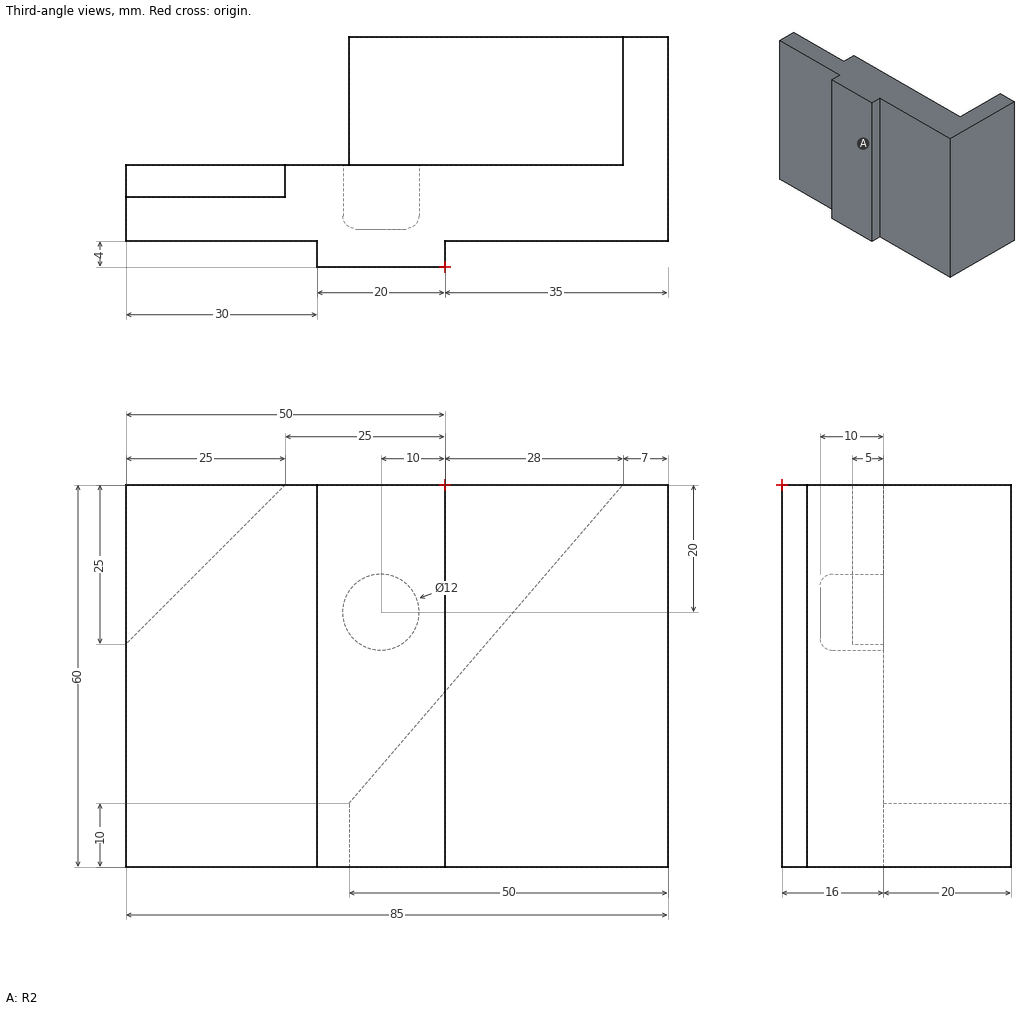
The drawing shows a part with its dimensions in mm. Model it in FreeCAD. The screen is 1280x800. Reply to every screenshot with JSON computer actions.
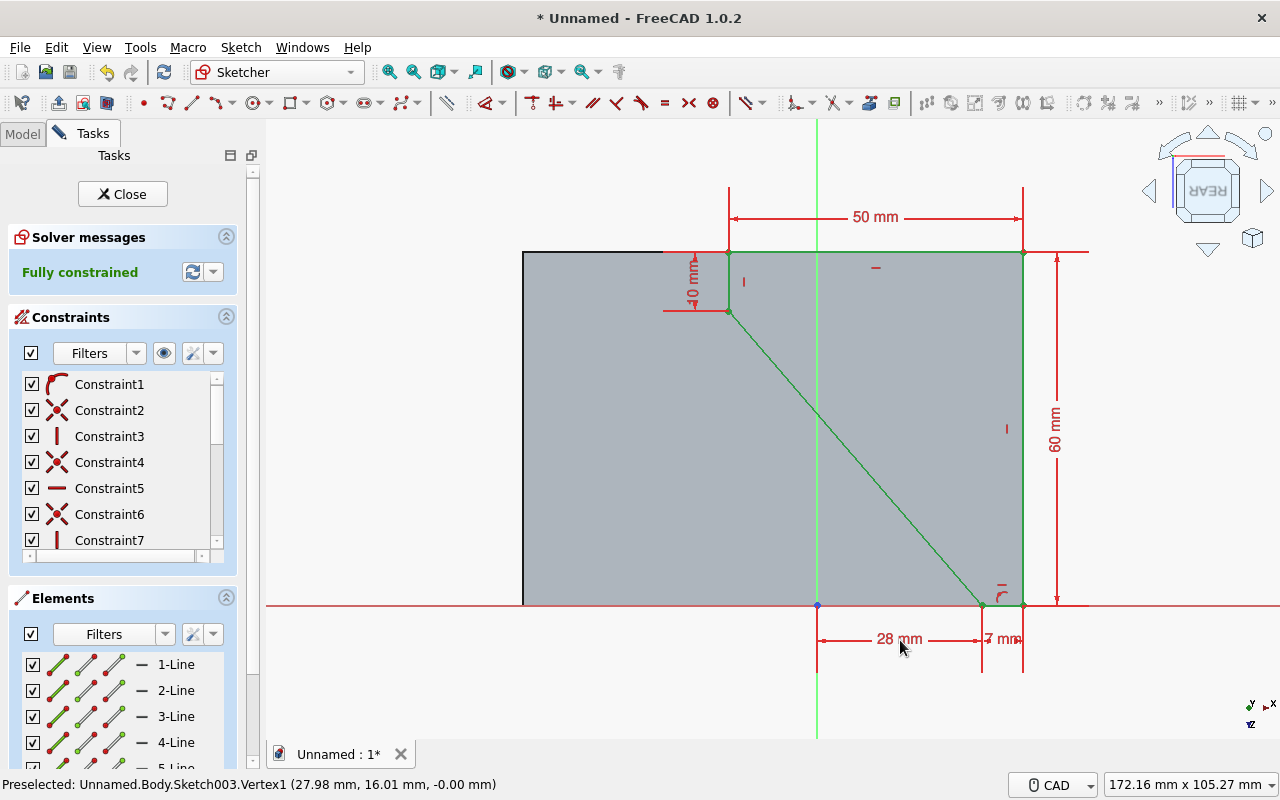
{"action": "left_click", "coordinate": [123, 194]}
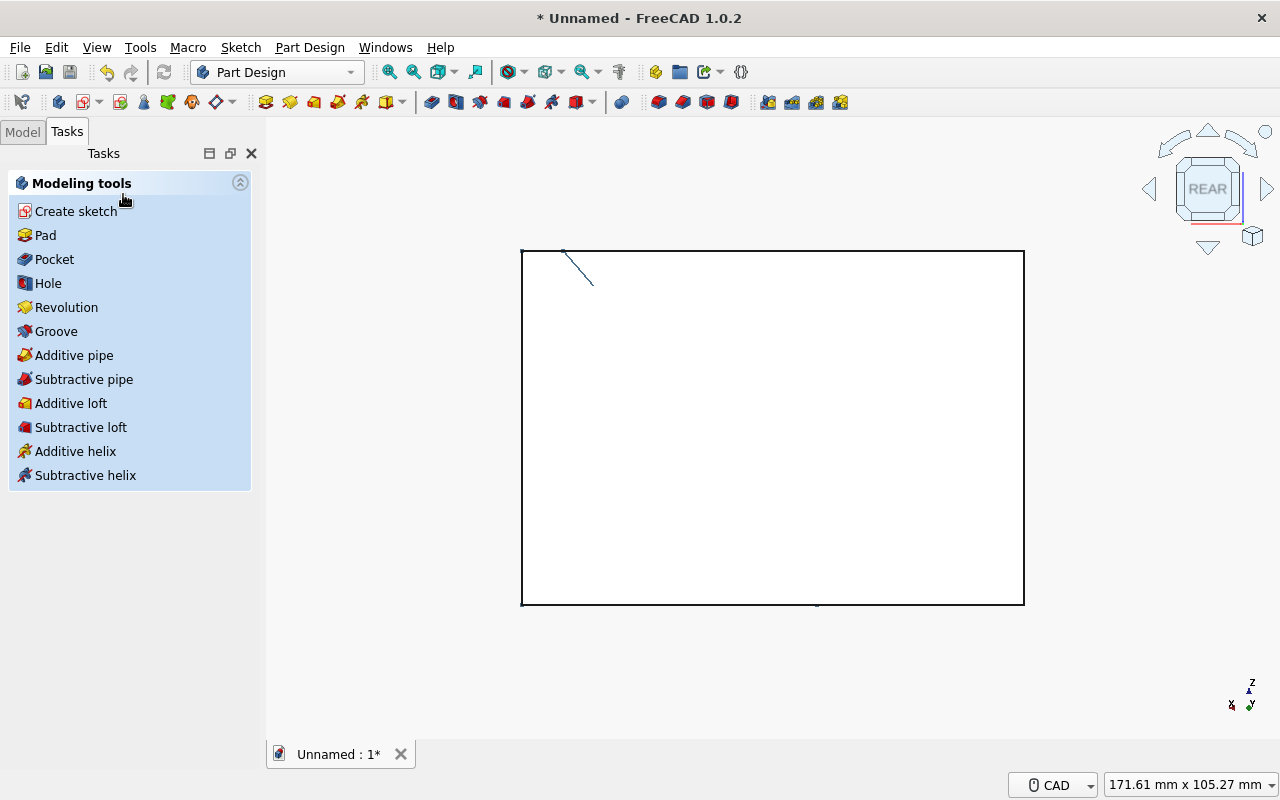
{"action": "left_click", "coordinate": [266, 102]}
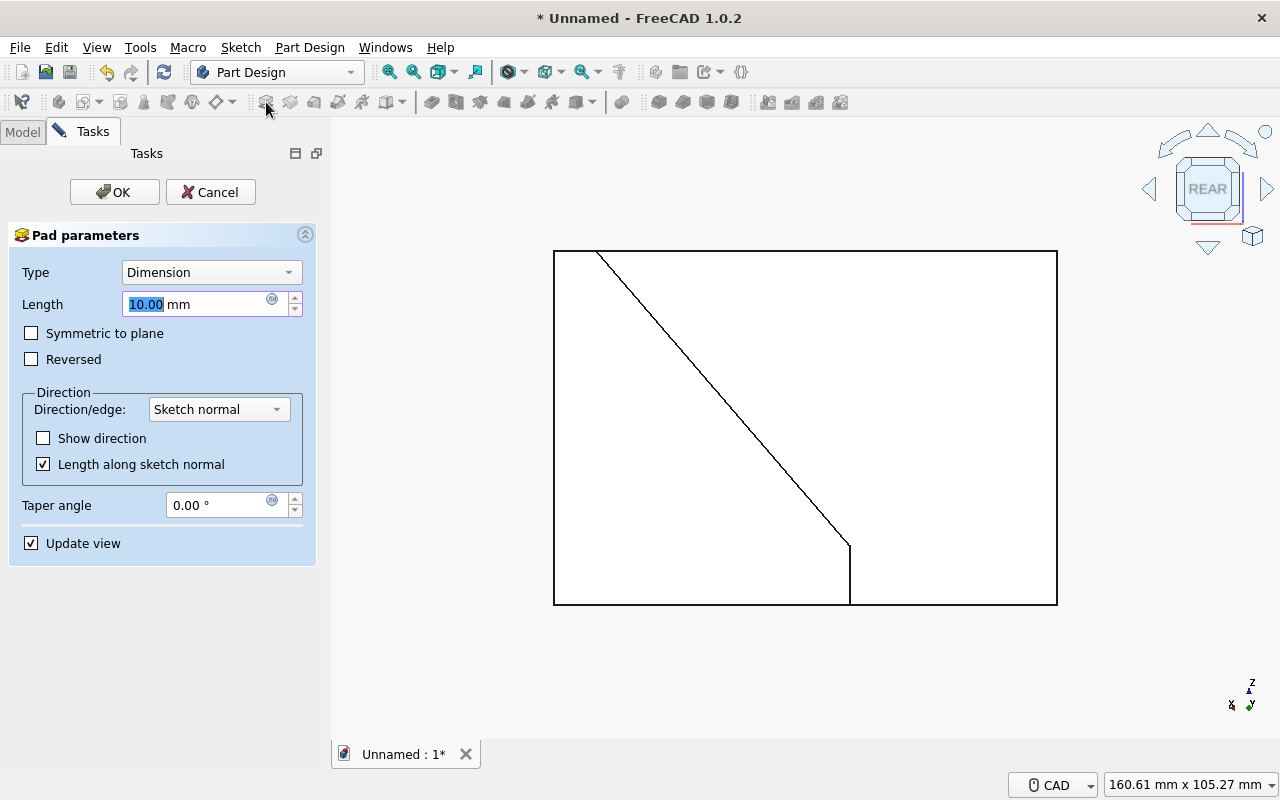
{"action": "type", "text": "20"}
{"action": "key", "text": "Tab"}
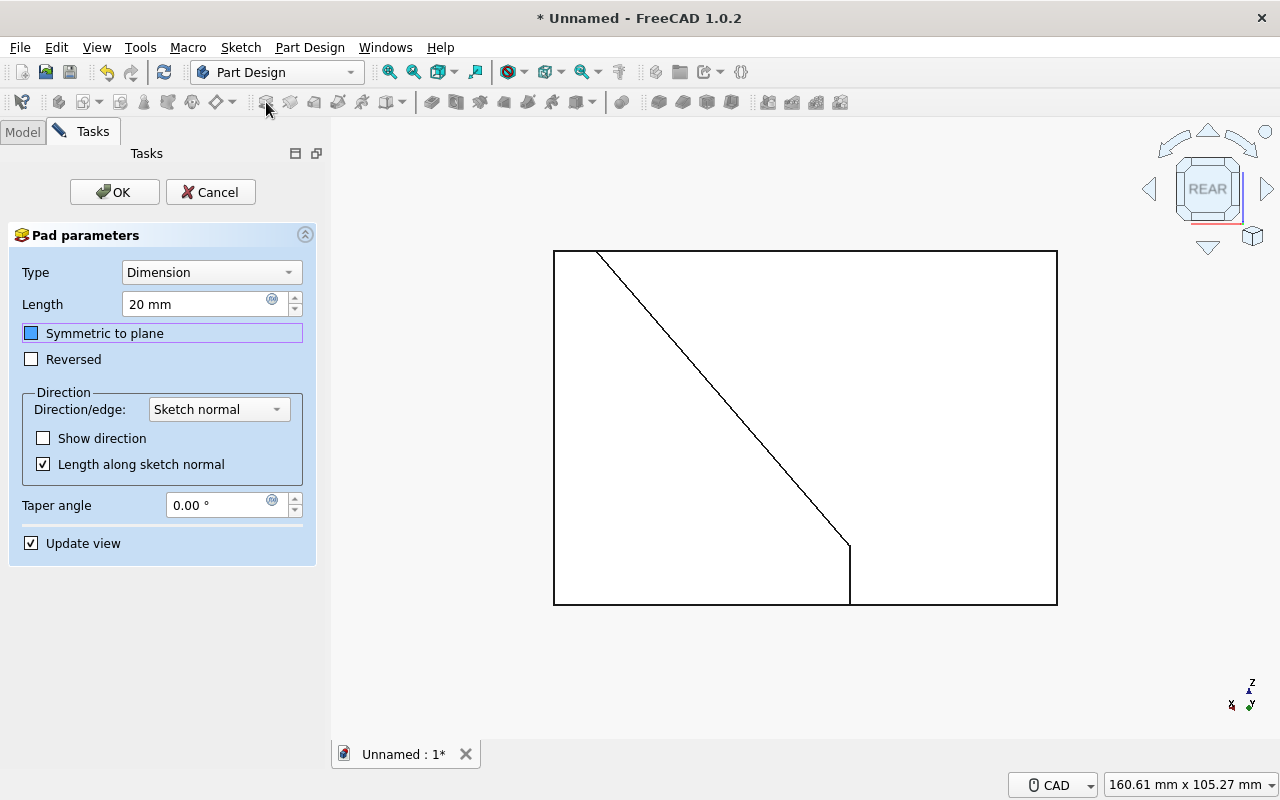
{"action": "left_click", "coordinate": [115, 192]}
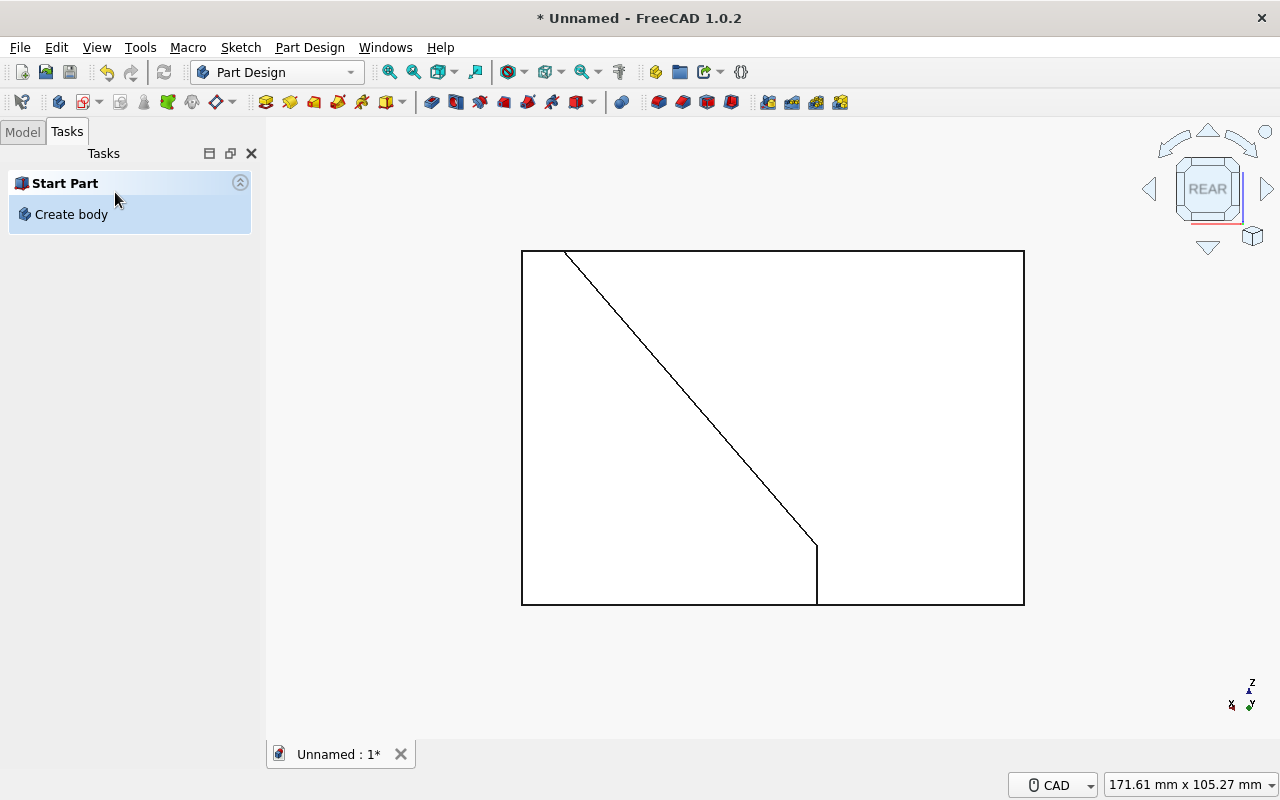
{"action": "left_click", "coordinate": [860, 376]}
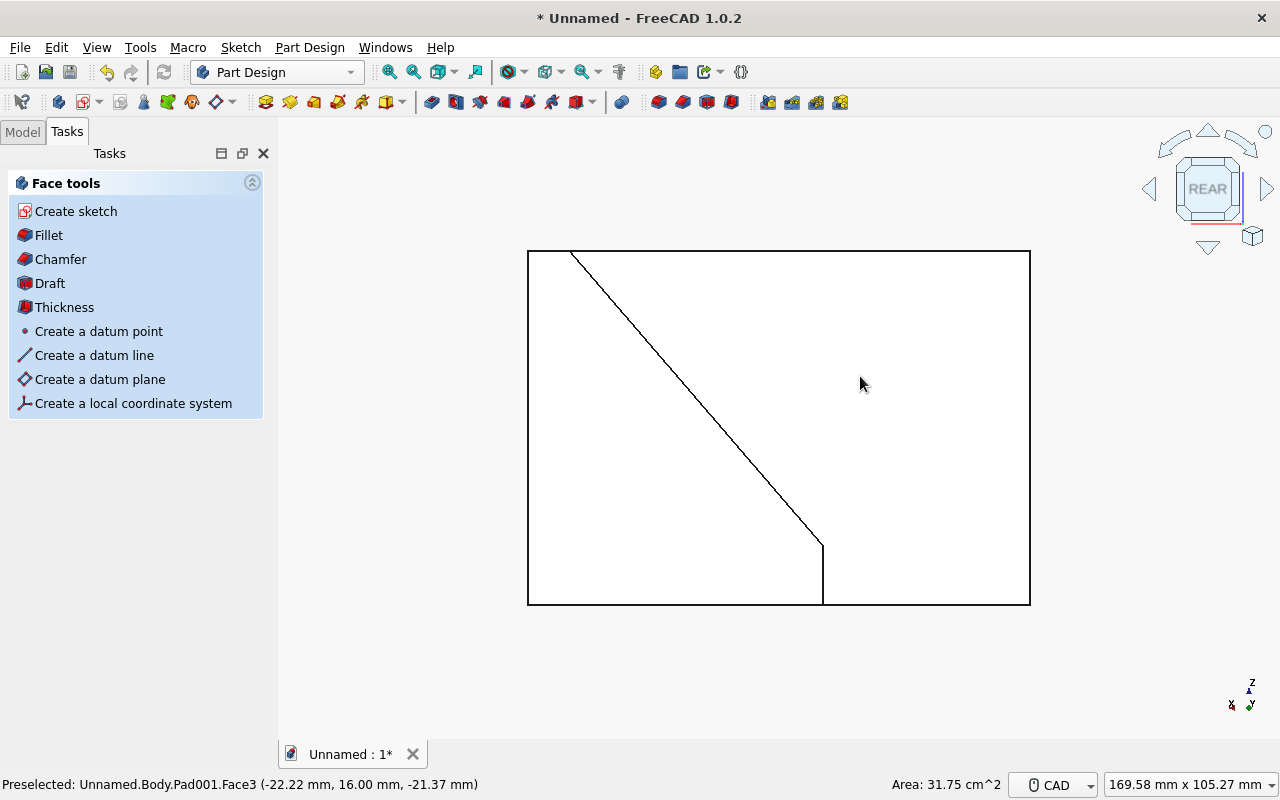
{"action": "left_click", "coordinate": [84, 102]}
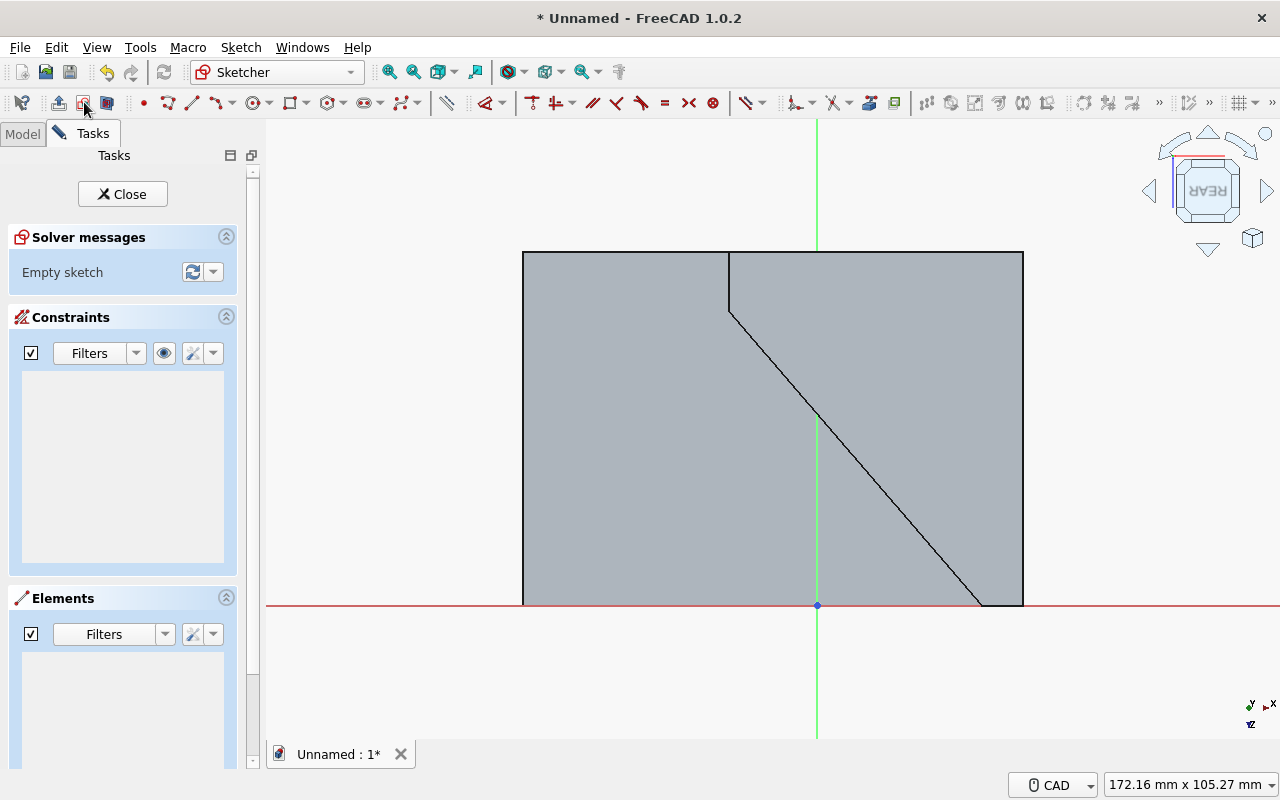
{"action": "left_click", "coordinate": [108, 104]}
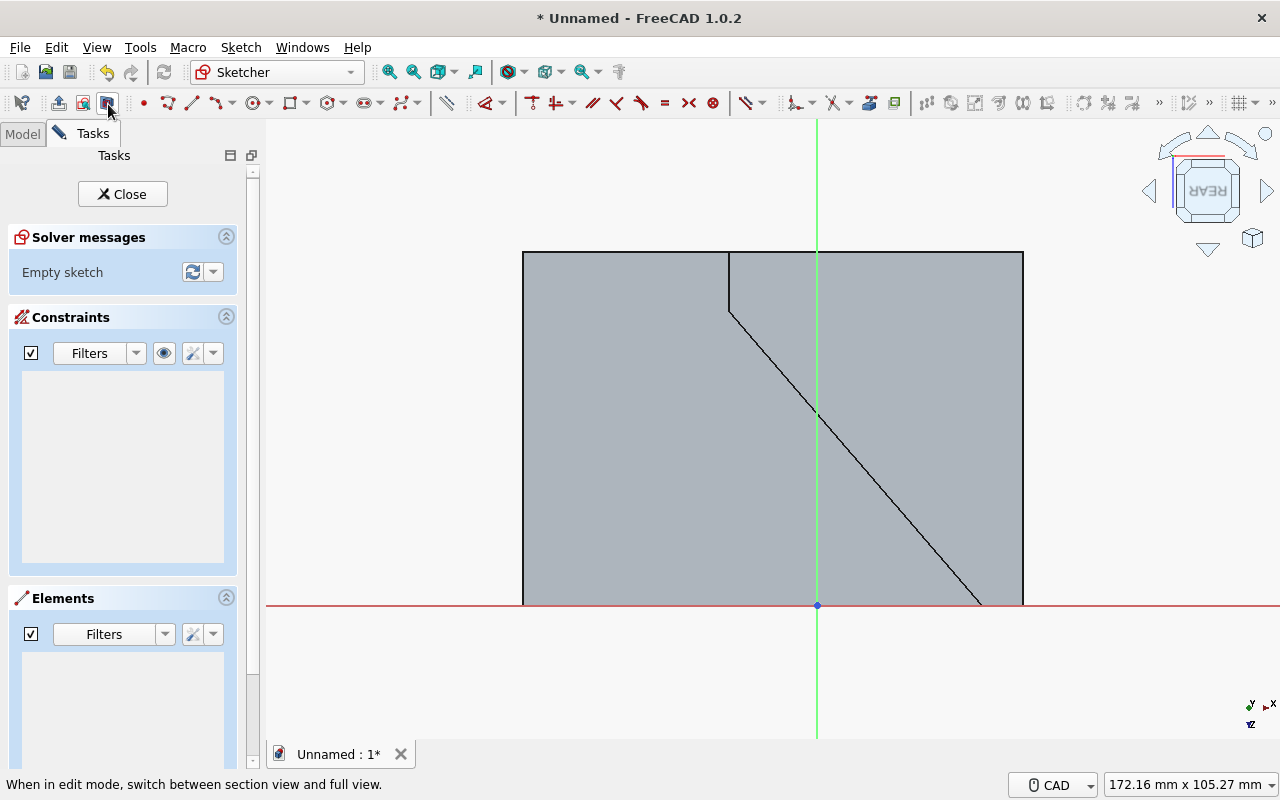
{"action": "scroll", "coordinate": [628, 657], "scroll_direction": "up", "scroll_amount": 3}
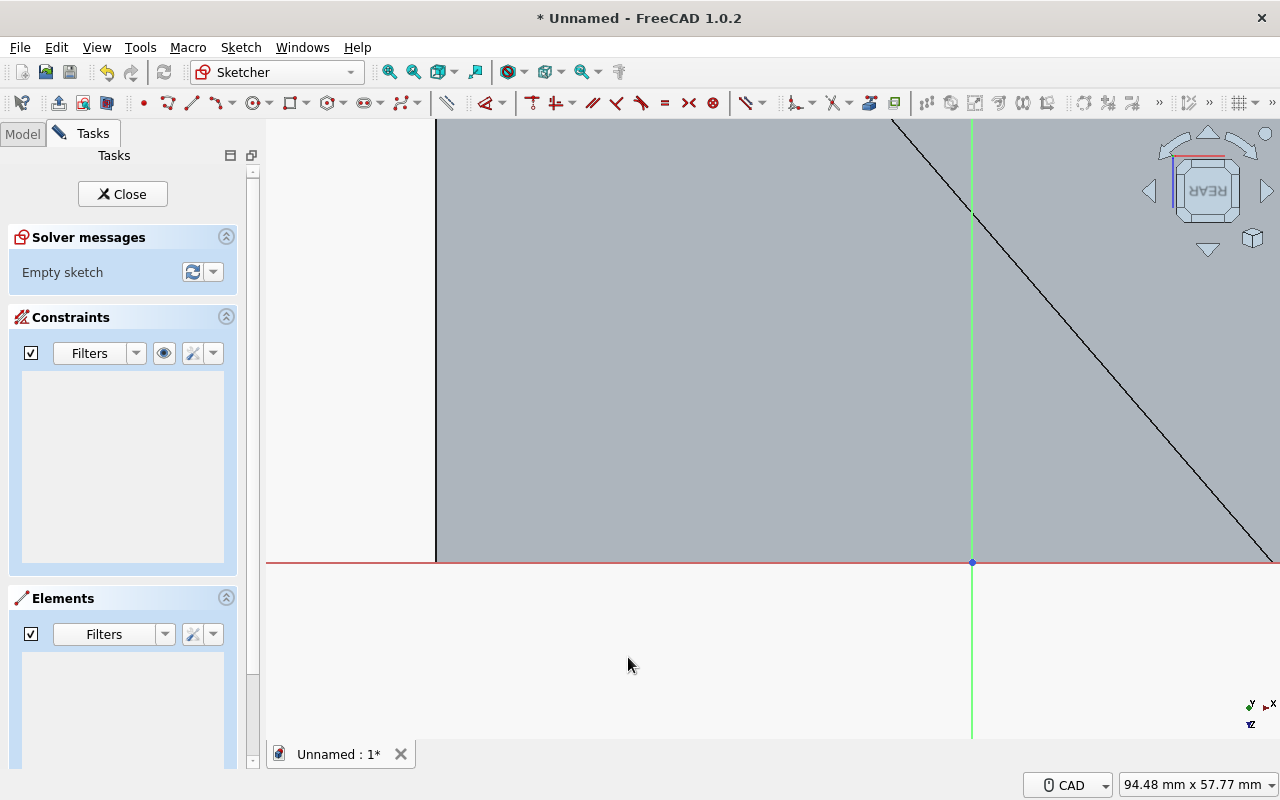
{"action": "left_click", "coordinate": [168, 104]}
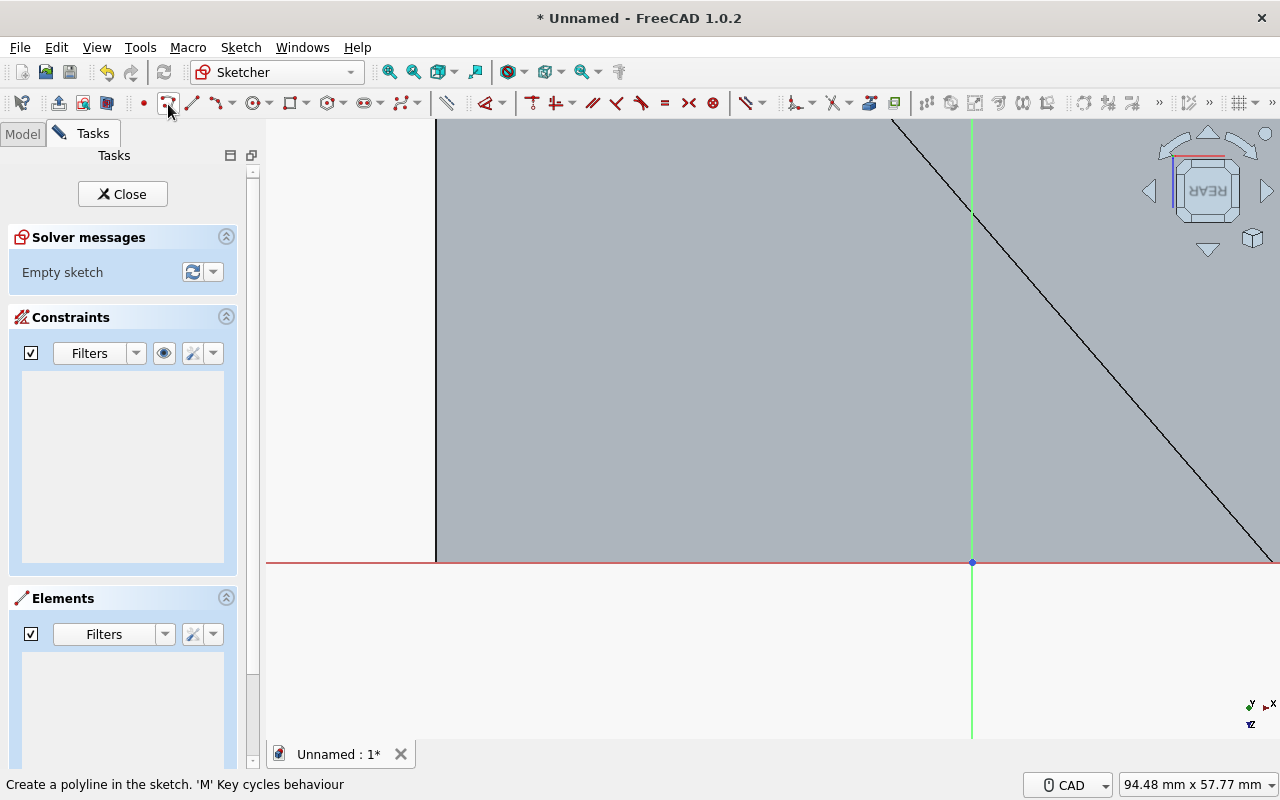
{"action": "left_click", "coordinate": [704, 563]}
{"action": "left_click", "coordinate": [436, 295]}
{"action": "left_click", "coordinate": [436, 554]}
{"action": "left_click", "coordinate": [704, 563]}
{"action": "key", "text": "Escape"}
{"action": "key", "text": "Escape"}